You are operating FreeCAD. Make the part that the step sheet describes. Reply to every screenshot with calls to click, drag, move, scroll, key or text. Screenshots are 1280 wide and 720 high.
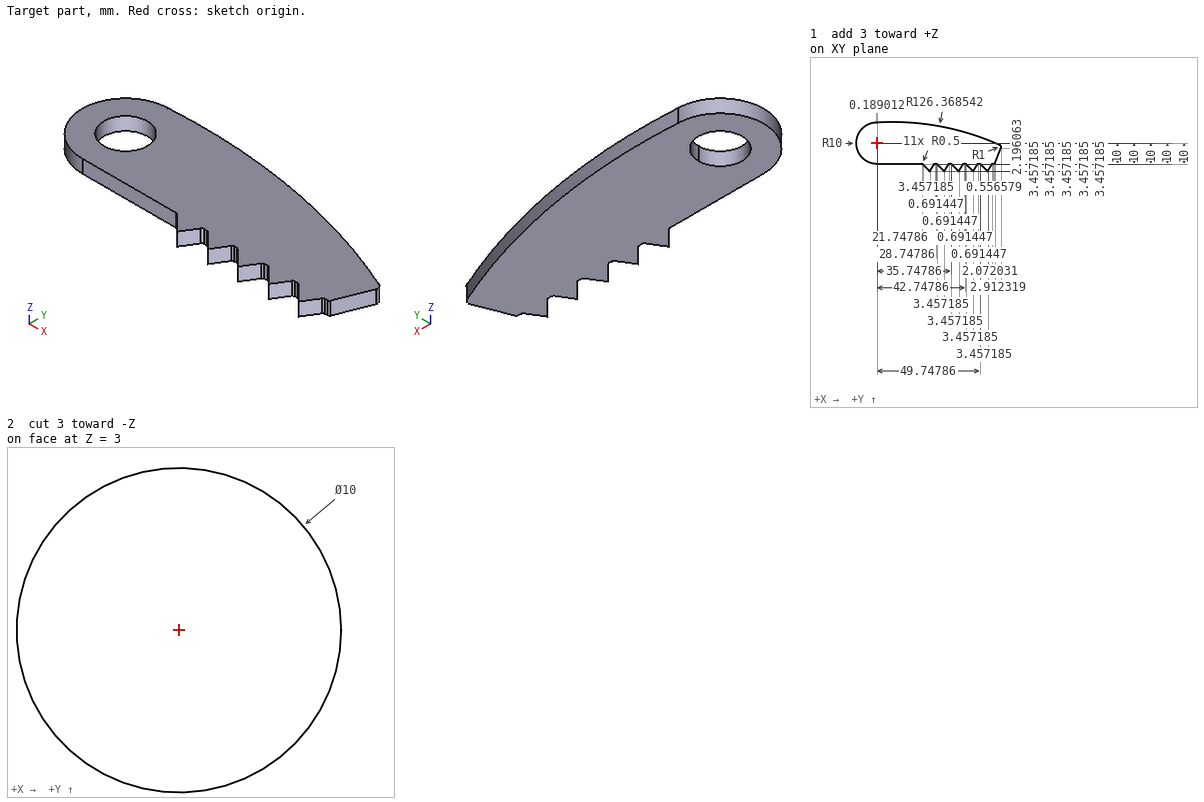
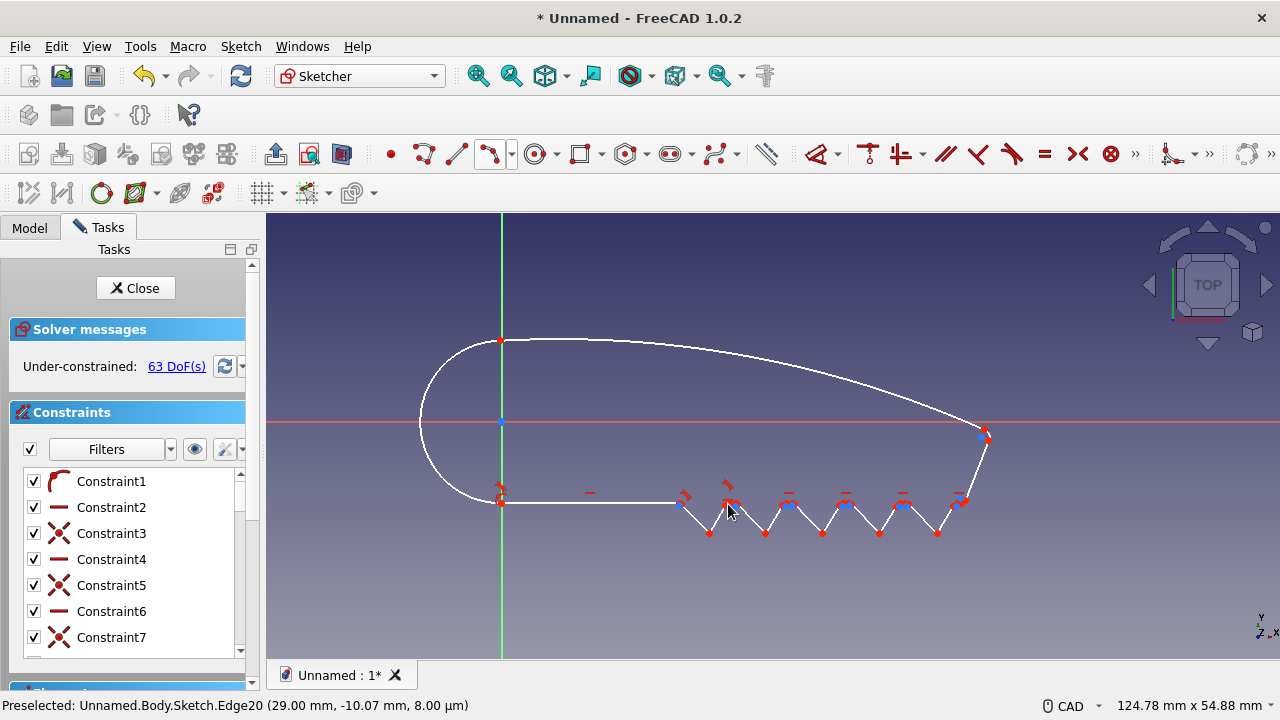
click(746, 513)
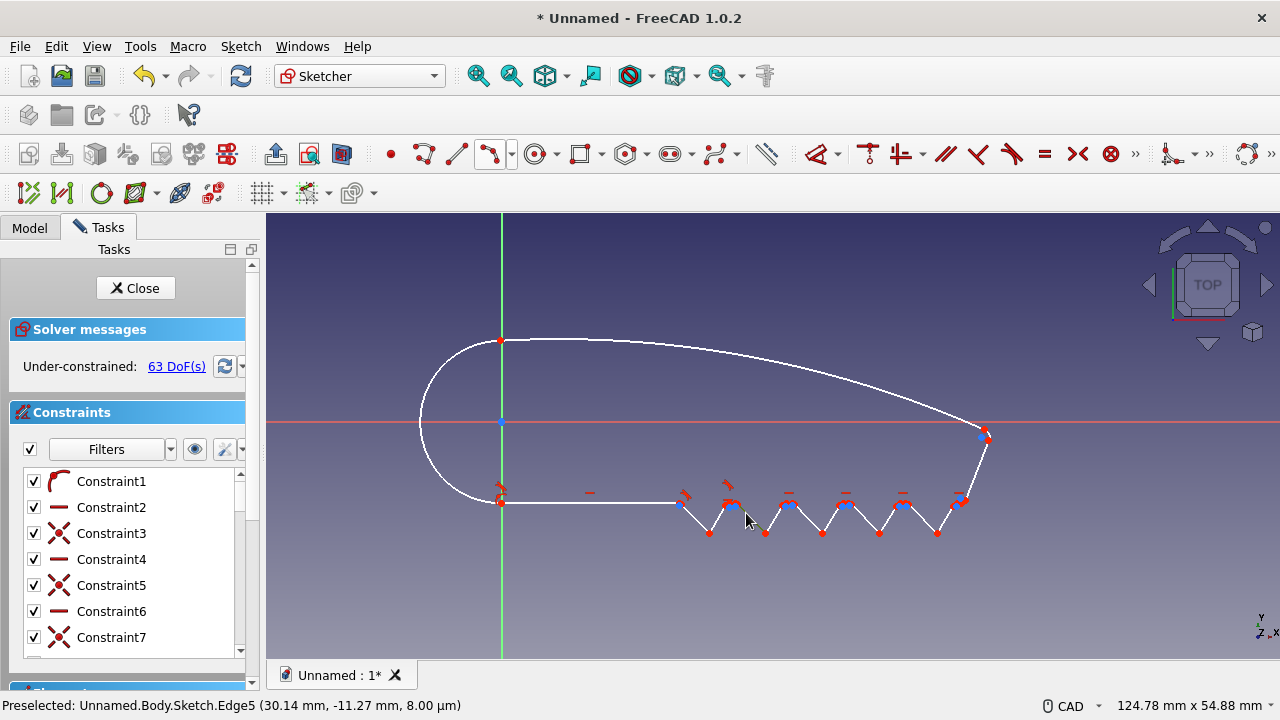
scroll(737, 504, up, 12)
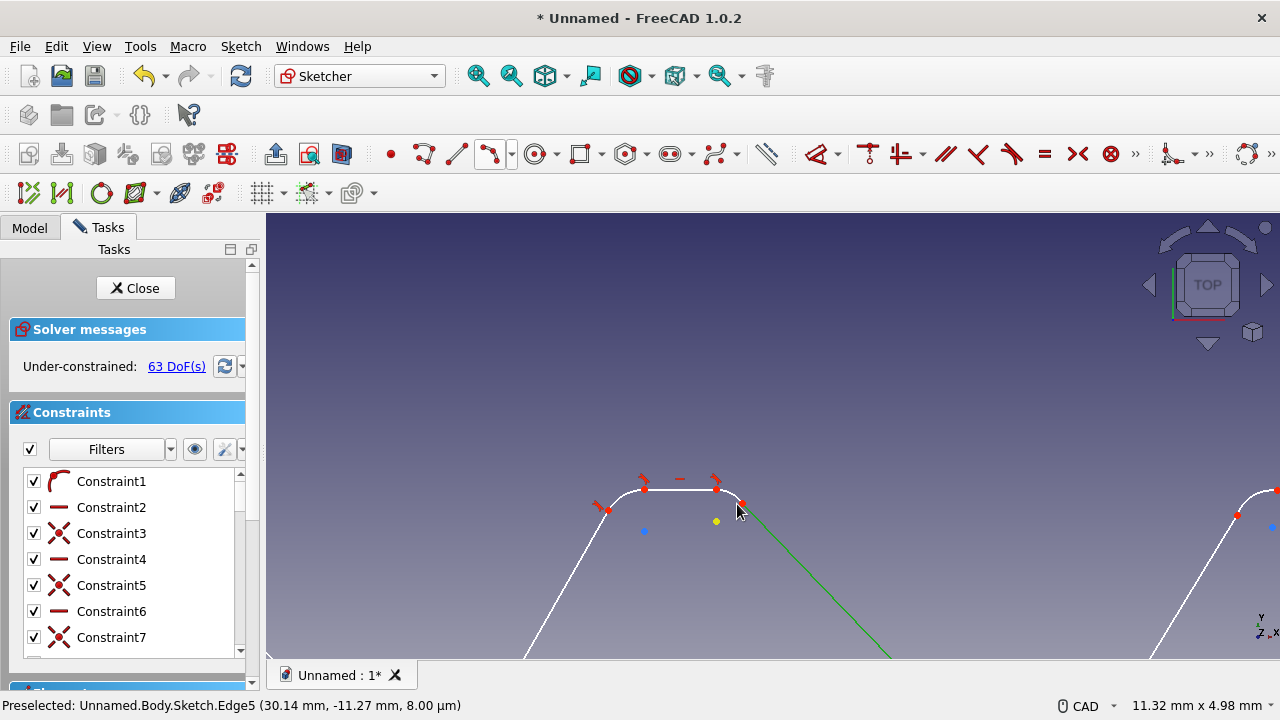
click(731, 493)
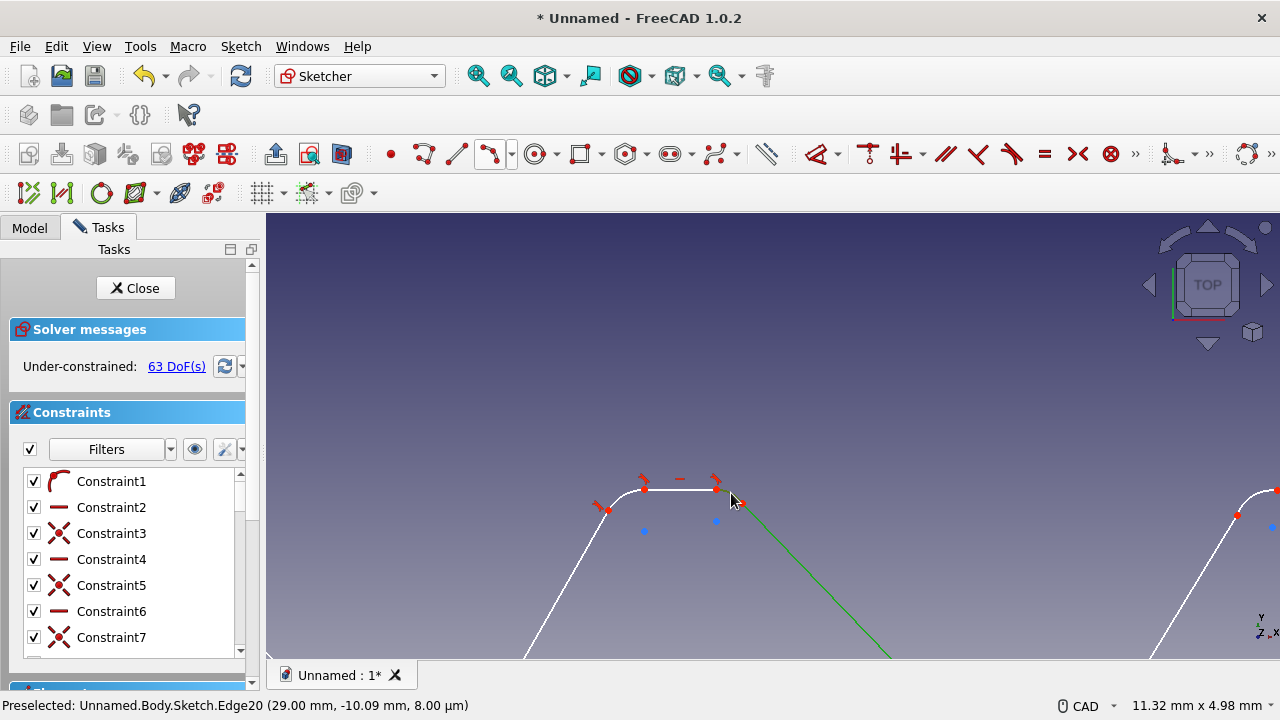
click(1012, 154)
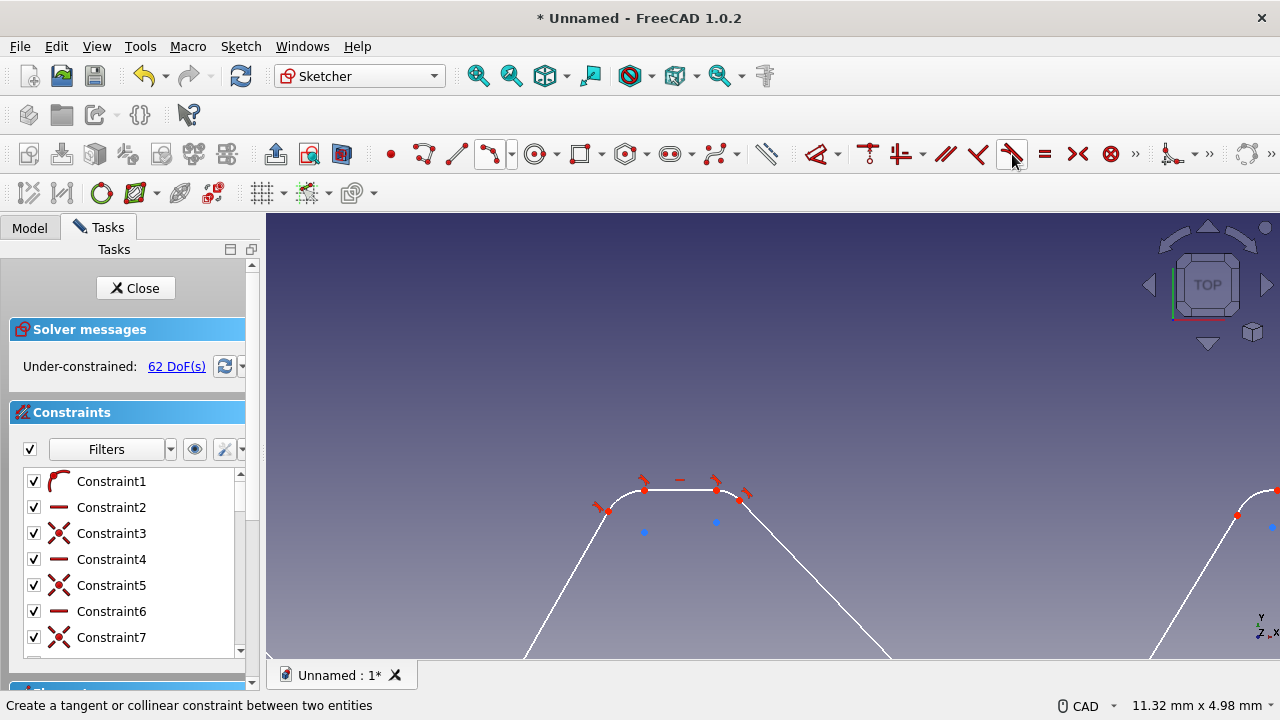
scroll(737, 504, down, 12)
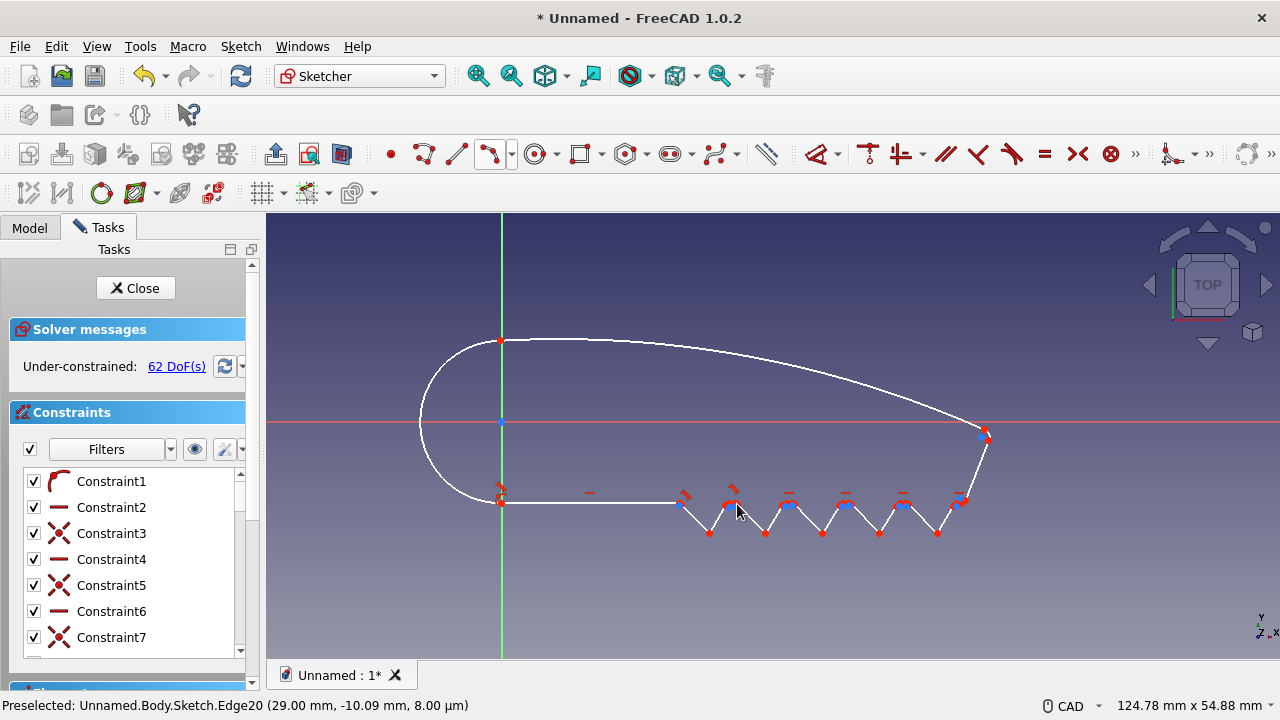
scroll(771, 525, up, 2)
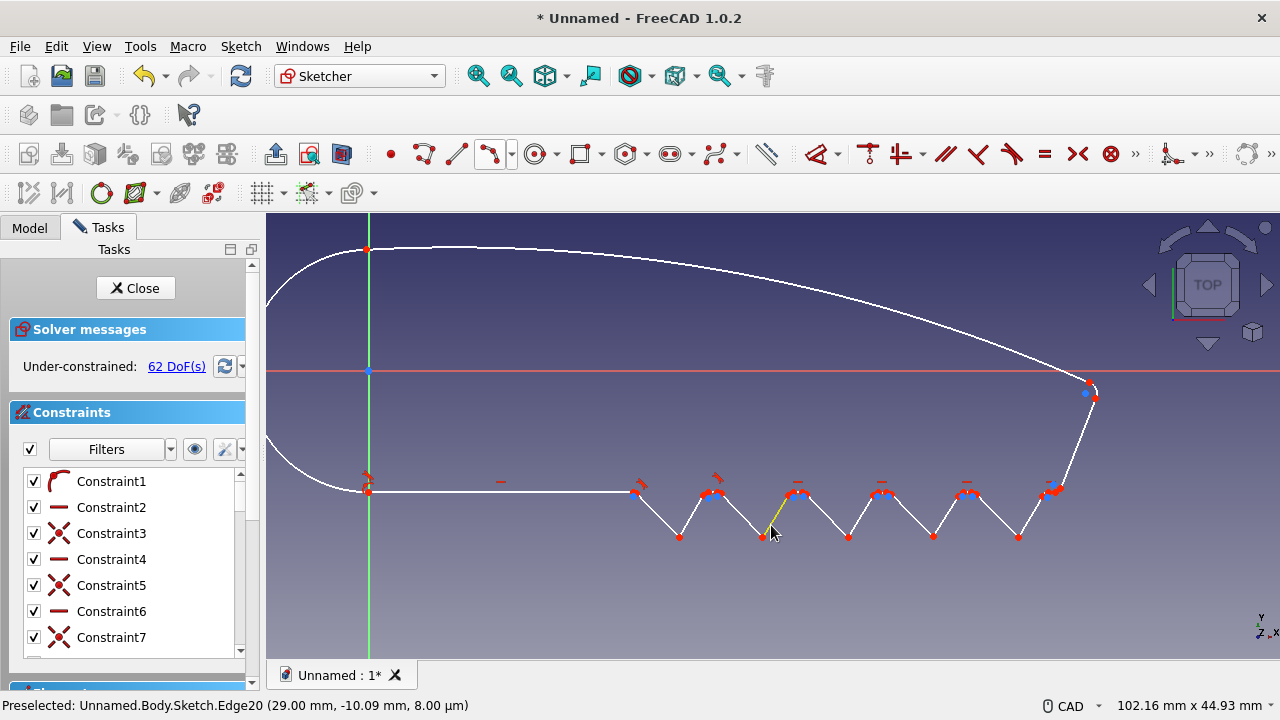
click(771, 525)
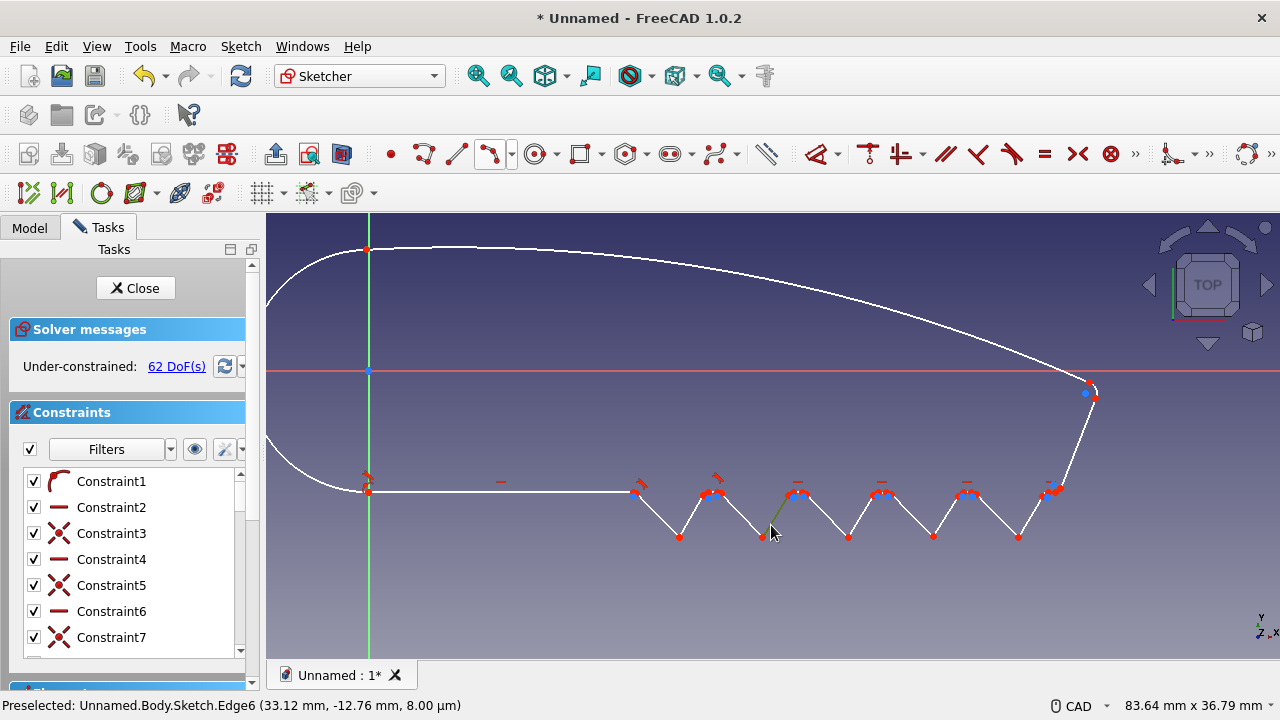
scroll(790, 493, up, 8)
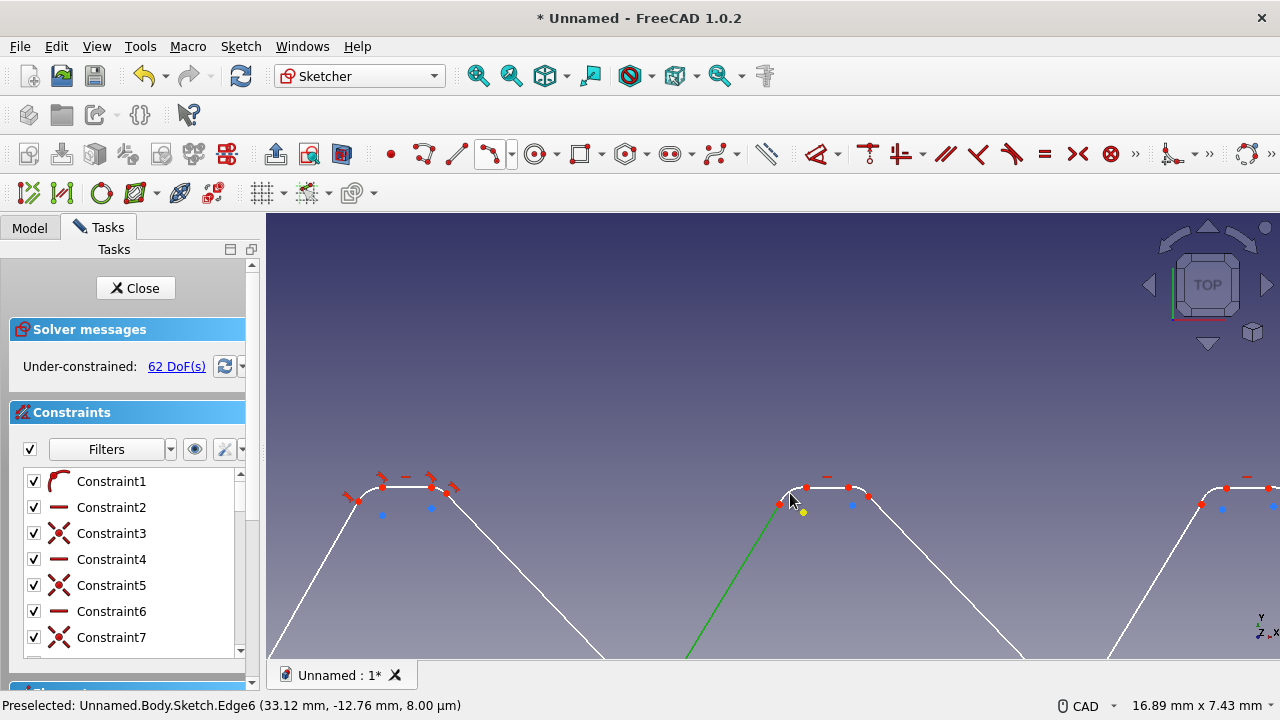
click(790, 491)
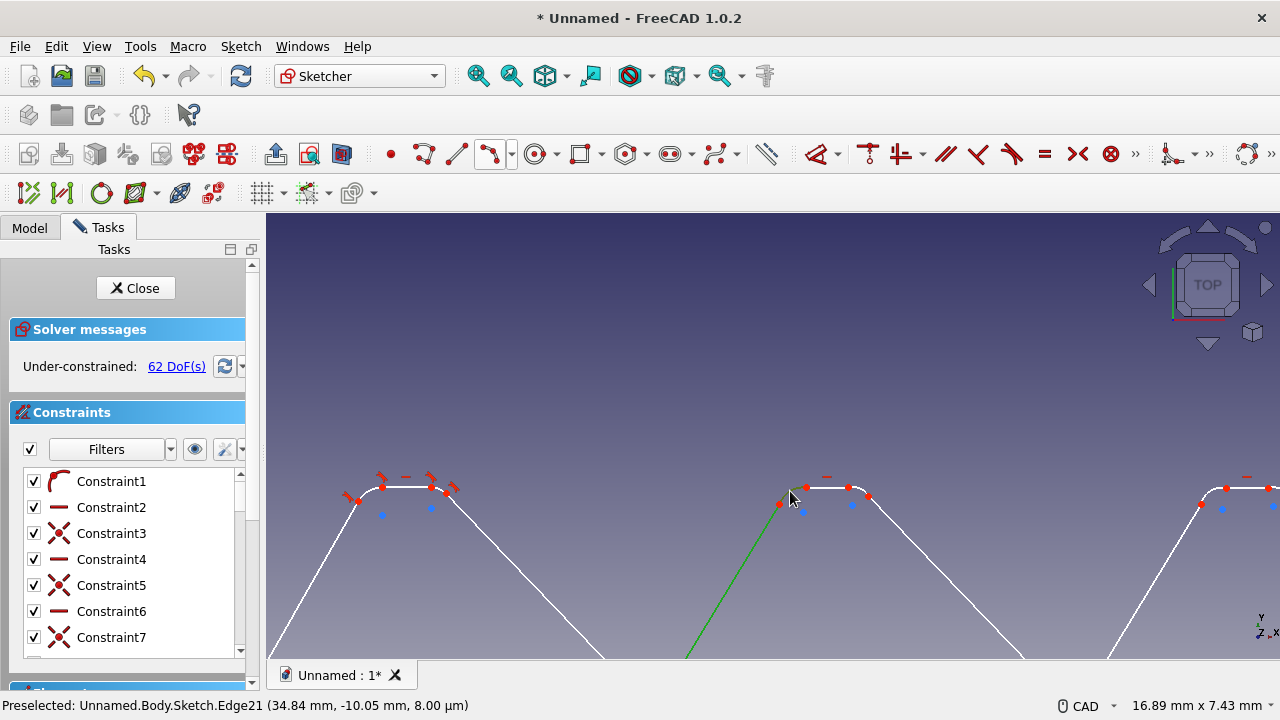
click(1012, 154)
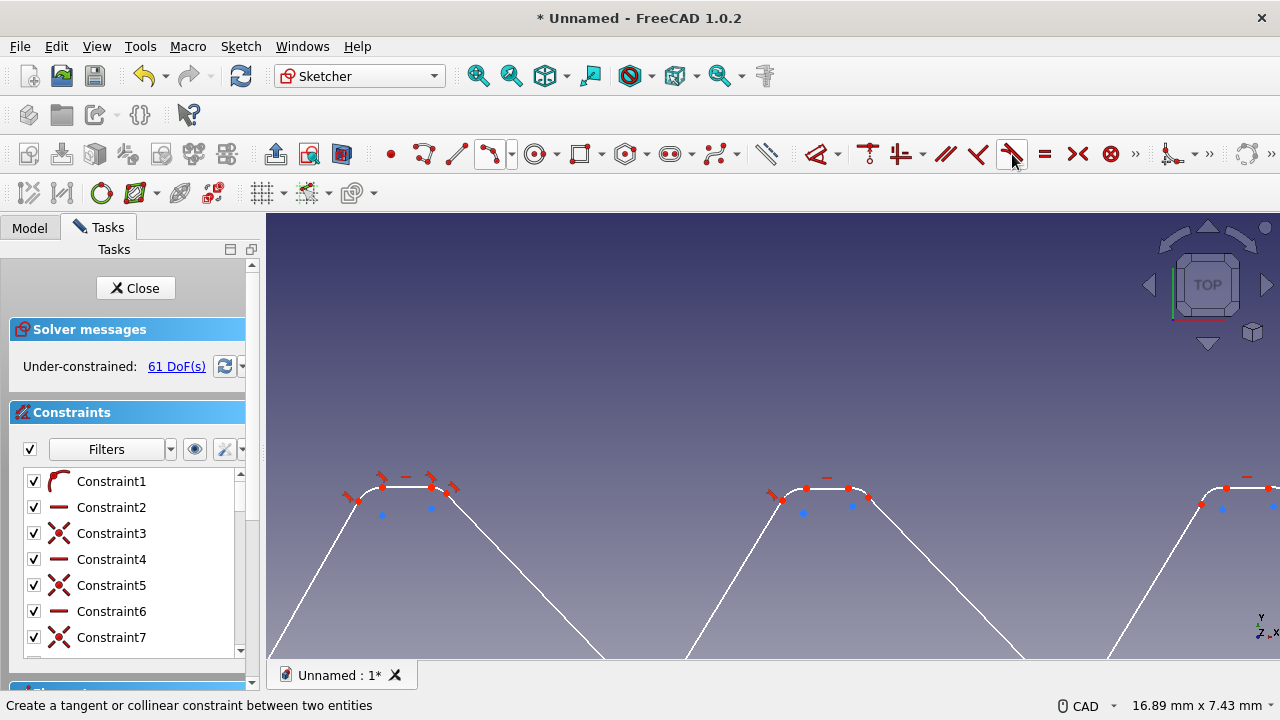
click(819, 489)